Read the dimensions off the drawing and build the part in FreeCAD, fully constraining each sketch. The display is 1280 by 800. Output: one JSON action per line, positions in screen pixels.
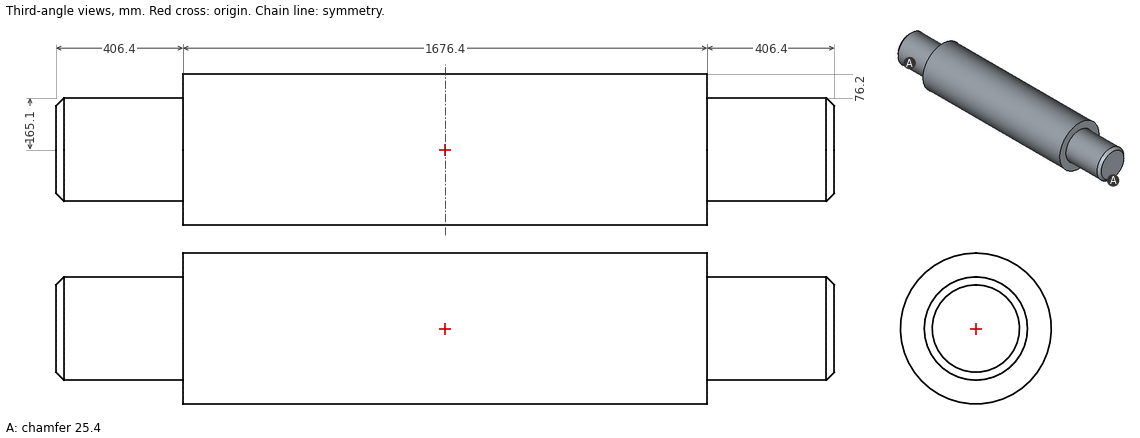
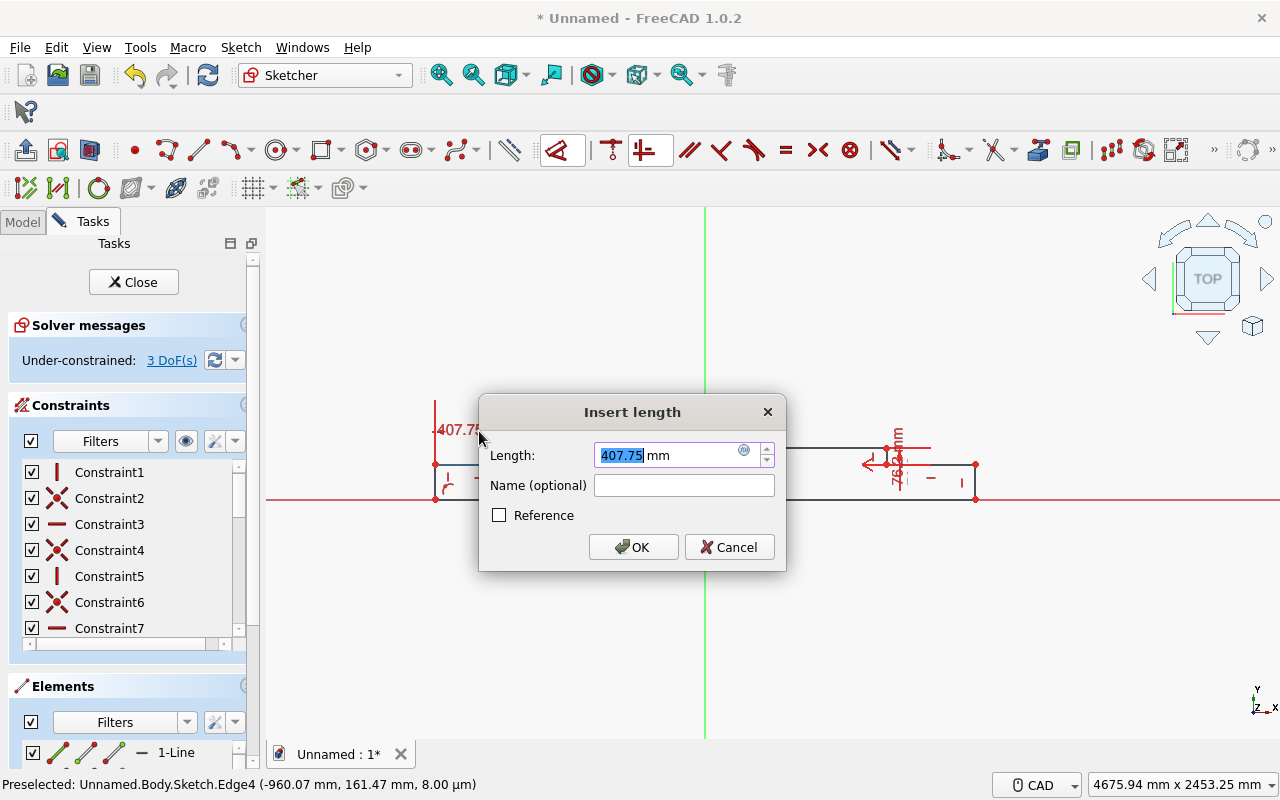
{"action": "type", "text": "406.4"}
{"action": "key", "text": "Return"}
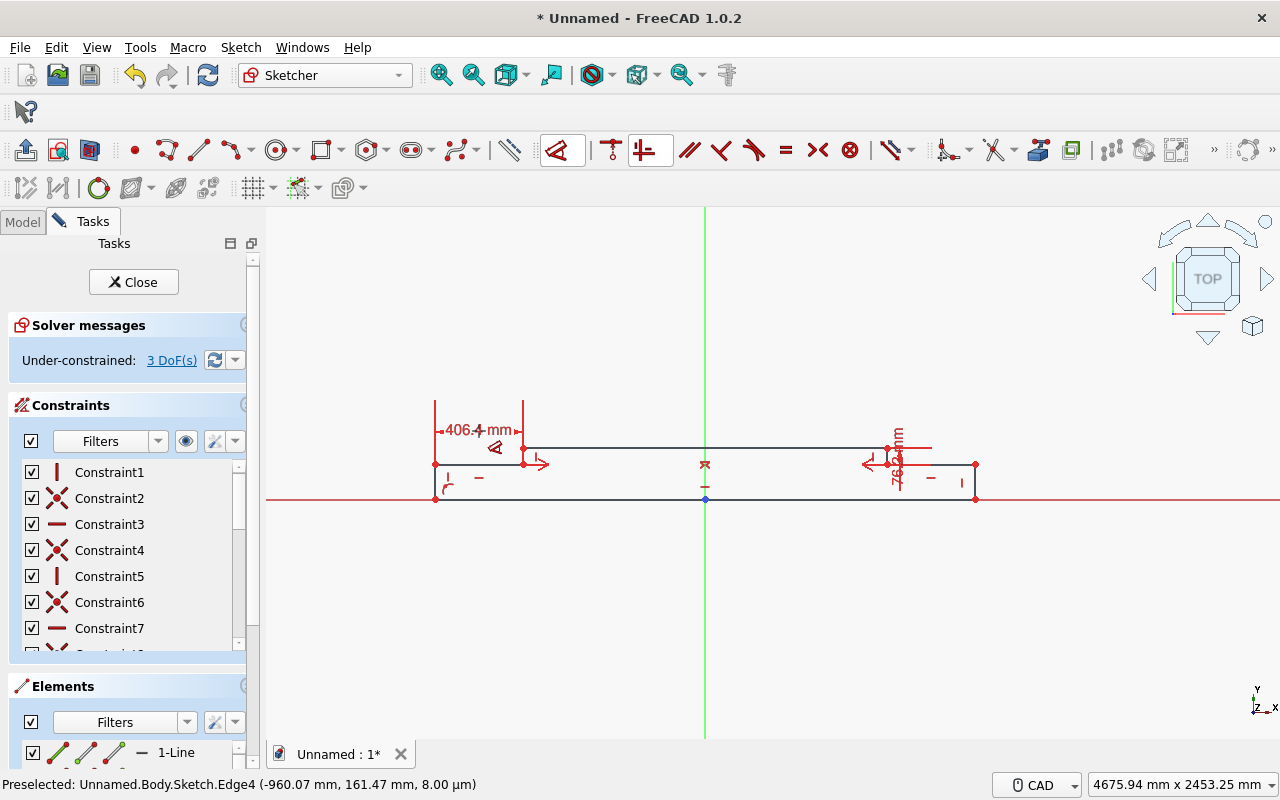
{"action": "scroll", "coordinate": [435, 475], "scroll_direction": "up", "scroll_amount": 2}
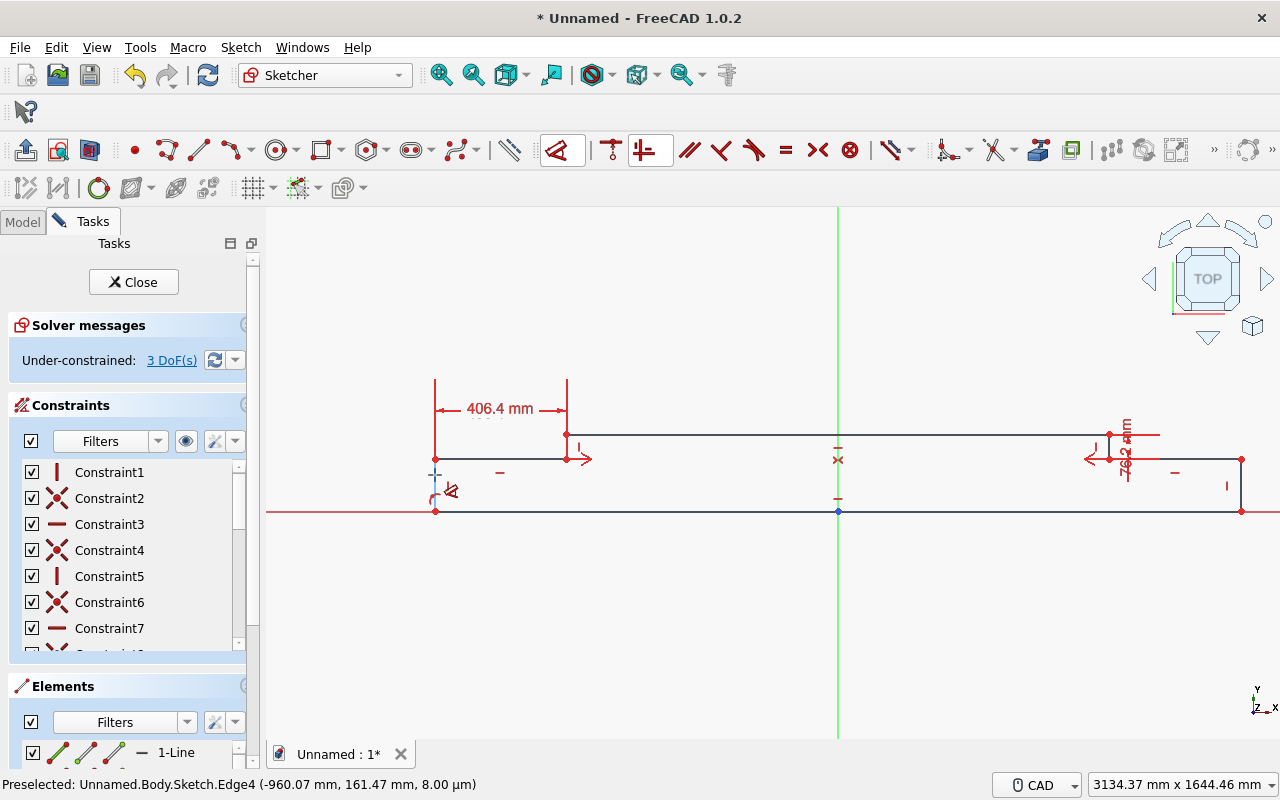
{"action": "left_click", "coordinate": [435, 475]}
{"action": "left_click", "coordinate": [401, 485]}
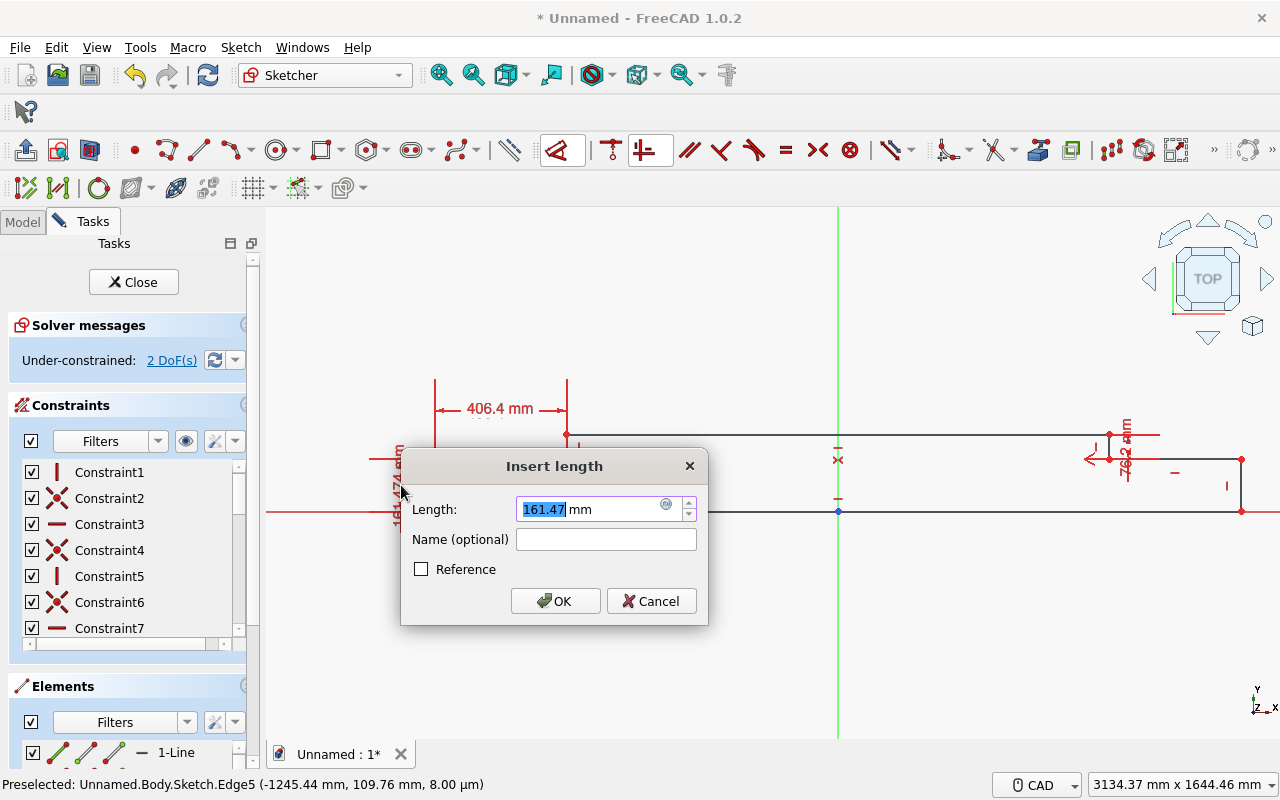
{"action": "type", "text": "165.1"}
{"action": "key", "text": "Return"}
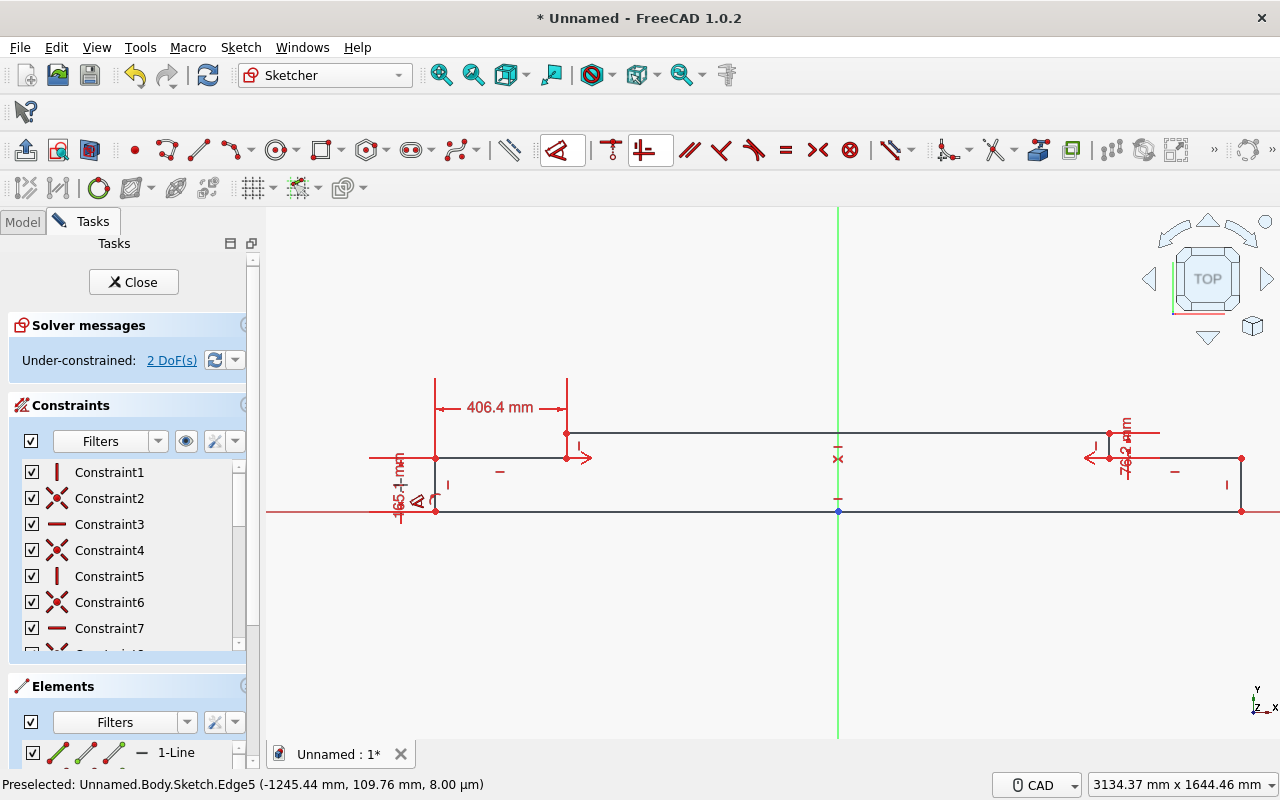
{"action": "scroll", "coordinate": [433, 474], "scroll_direction": "down", "scroll_amount": 2}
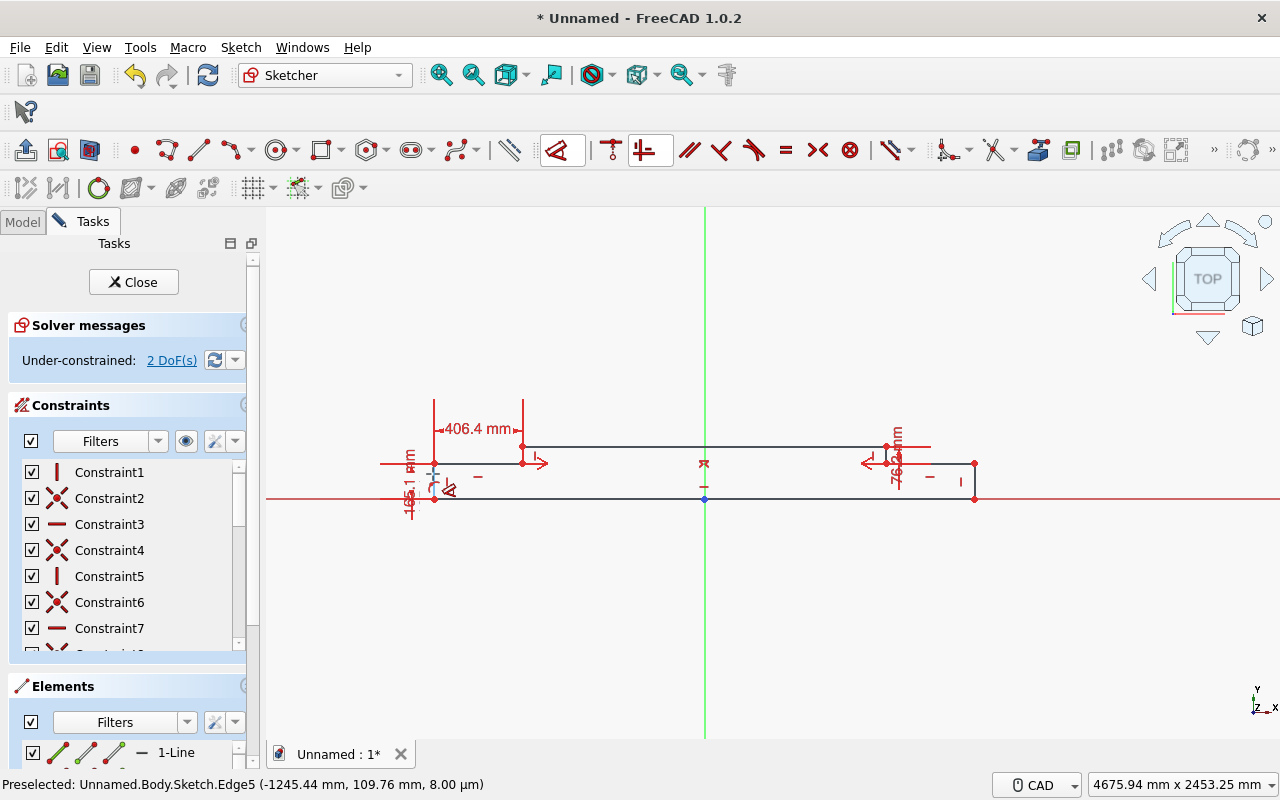
{"action": "left_click", "coordinate": [948, 464]}
{"action": "left_click", "coordinate": [931, 430]}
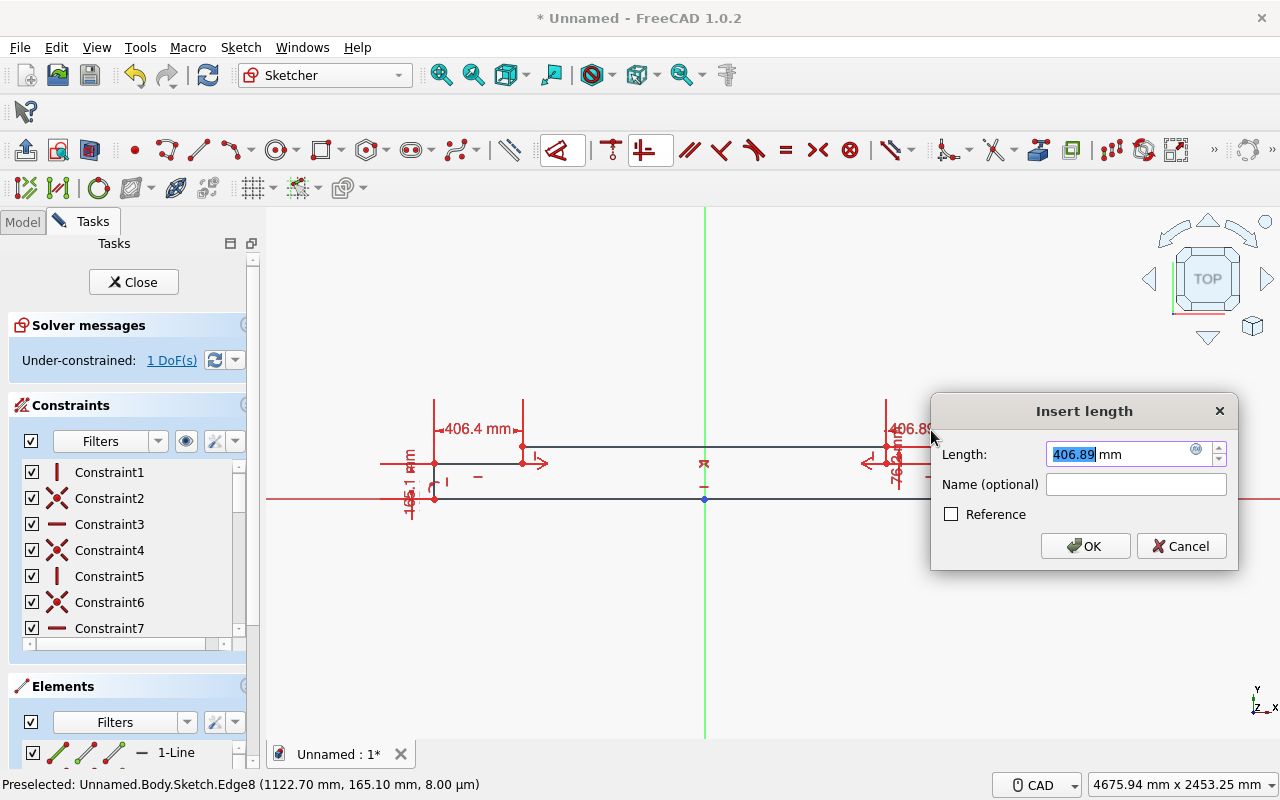
{"action": "type", "text": "406.4"}
{"action": "key", "text": "Return"}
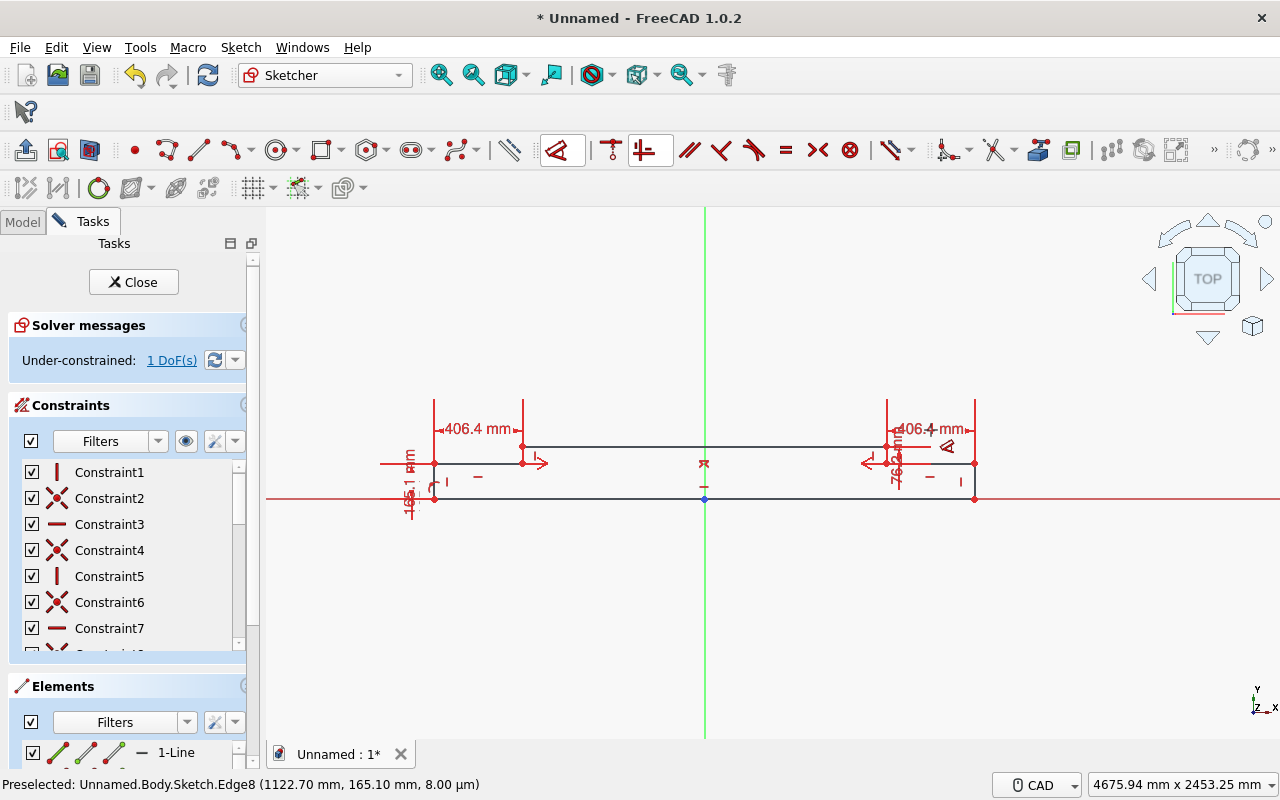
{"action": "left_click", "coordinate": [777, 447]}
{"action": "left_click", "coordinate": [621, 413]}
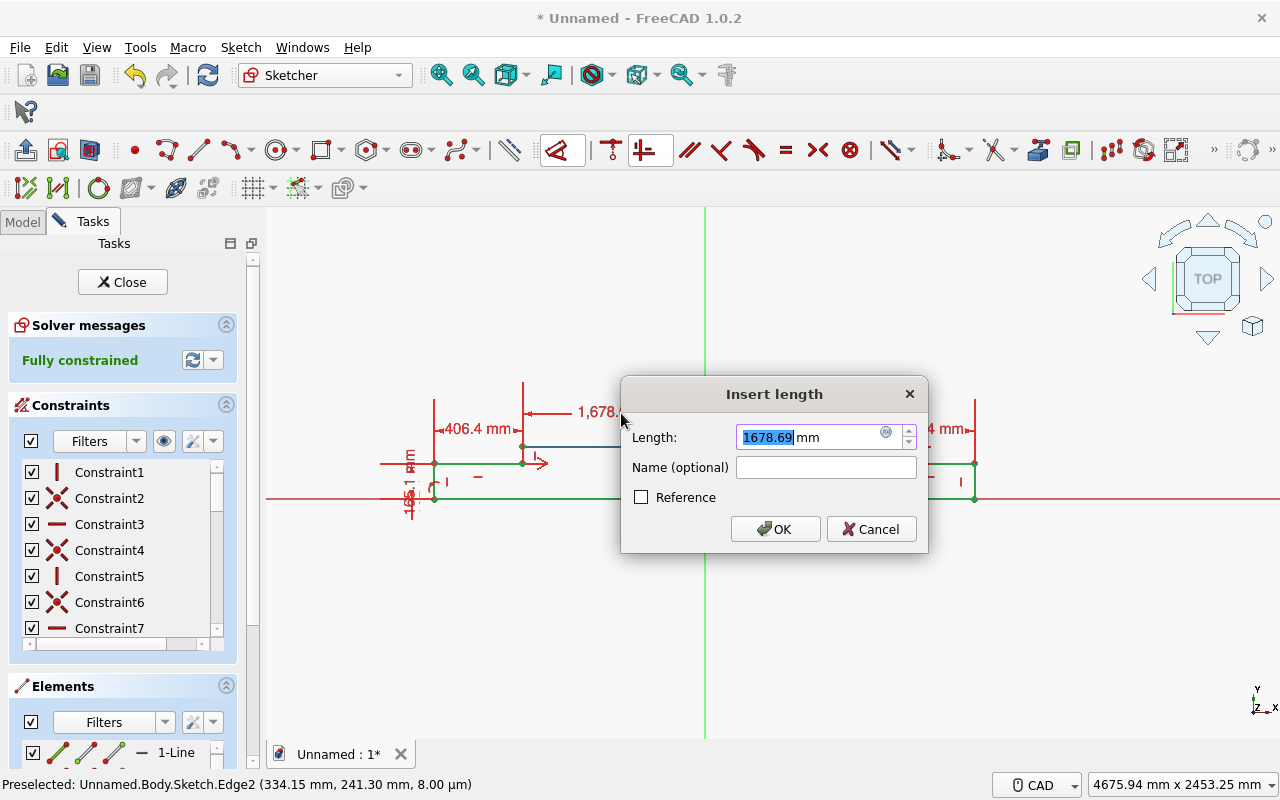
{"action": "type", "text": "1676.4"}
{"action": "key", "text": "Return"}
{"action": "key", "text": "Escape"}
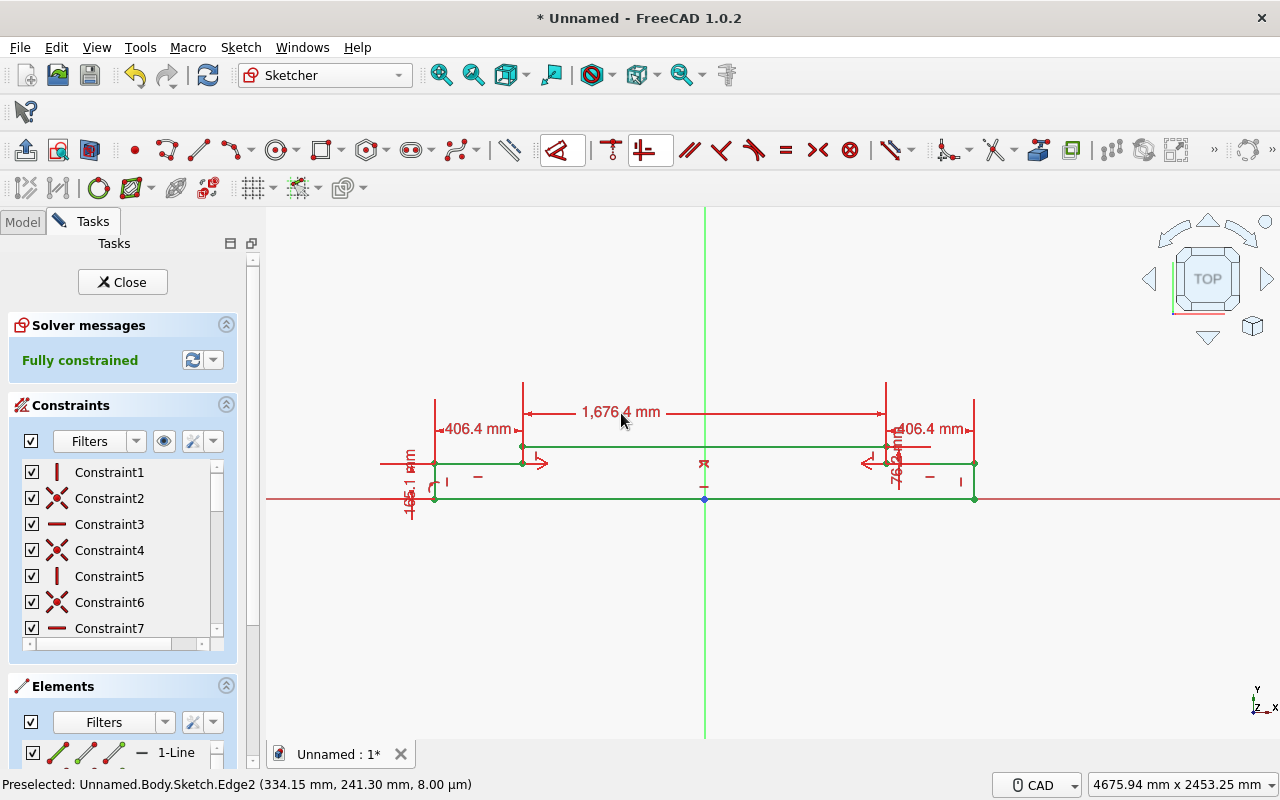
{"action": "left_click", "coordinate": [123, 282]}